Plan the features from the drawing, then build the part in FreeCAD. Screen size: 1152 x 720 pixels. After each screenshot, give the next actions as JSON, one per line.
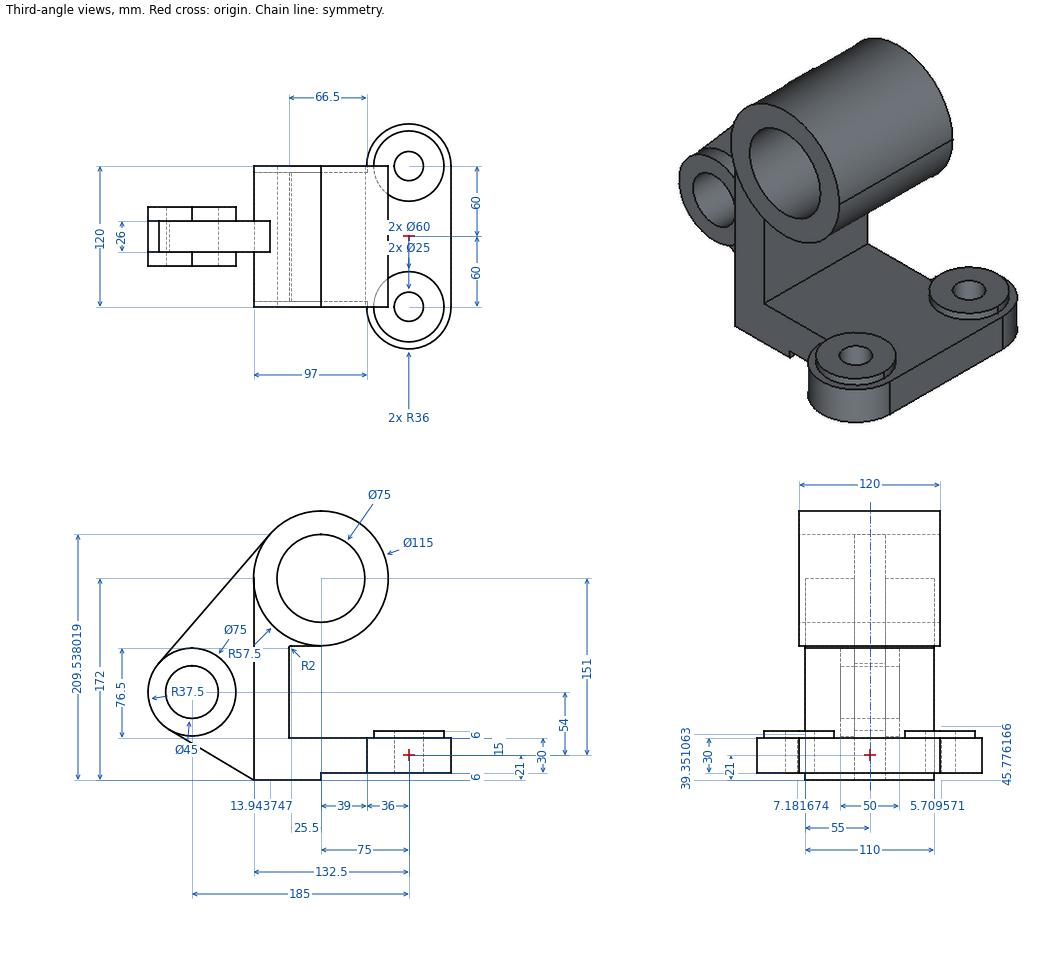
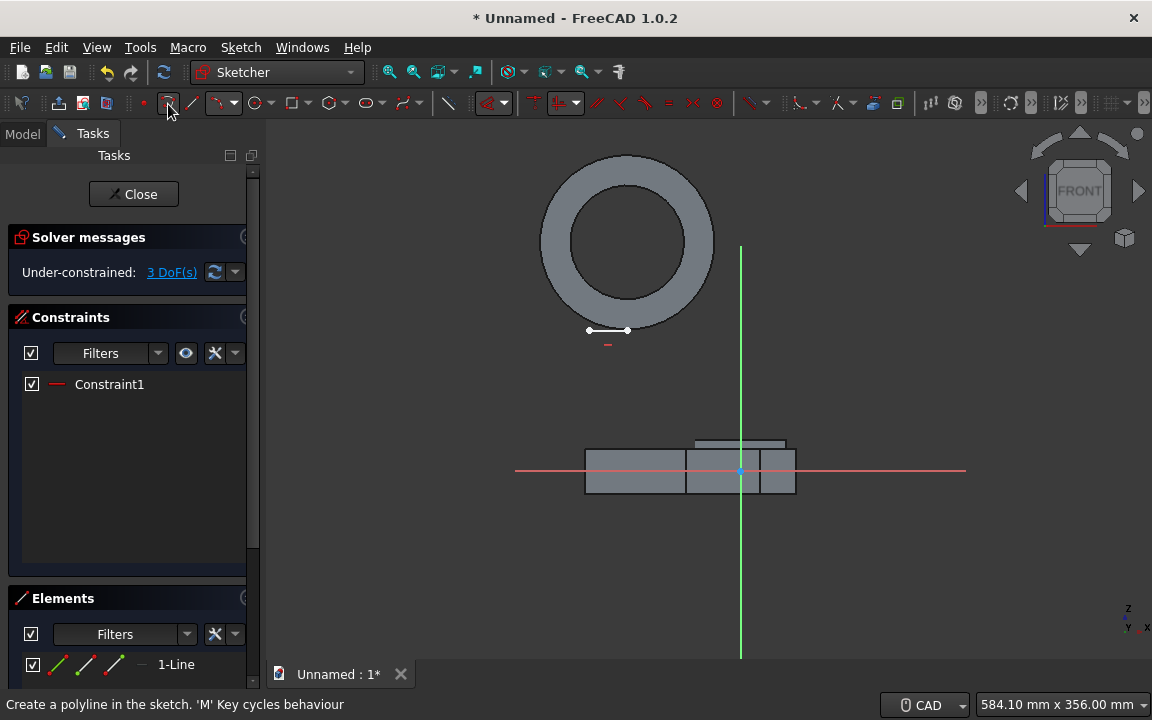
{"action": "scroll", "coordinate": [586, 333], "scroll_direction": "up", "scroll_amount": 7}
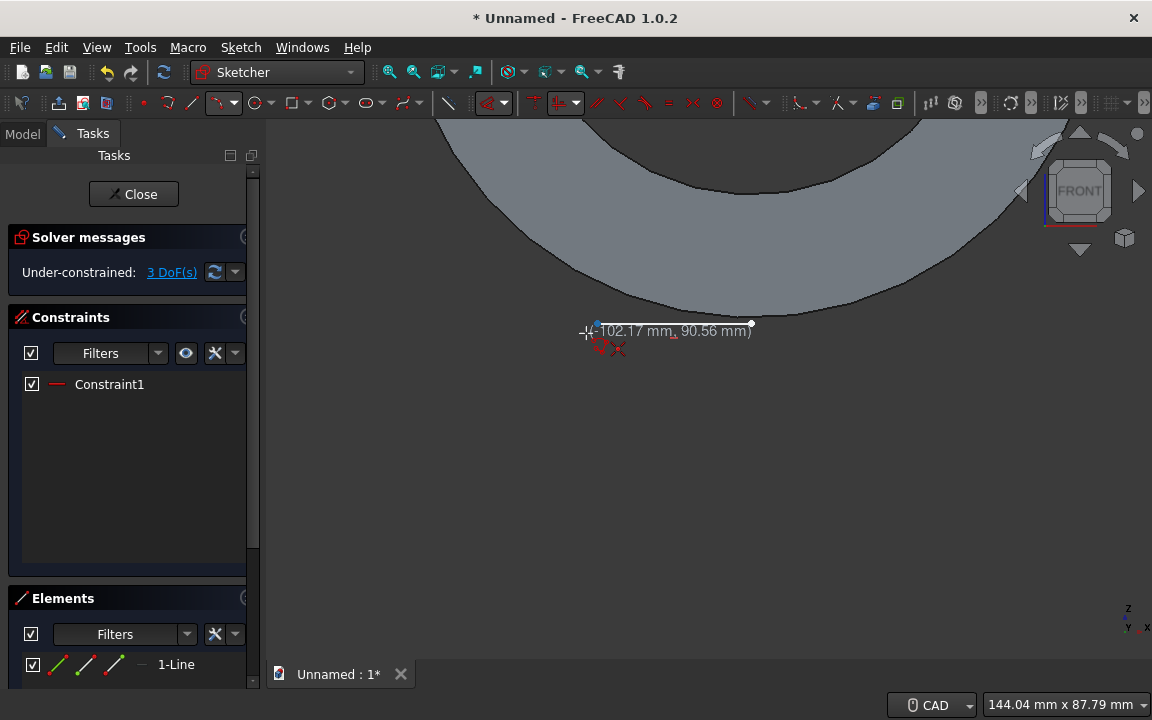
{"action": "left_click", "coordinate": [583, 330]}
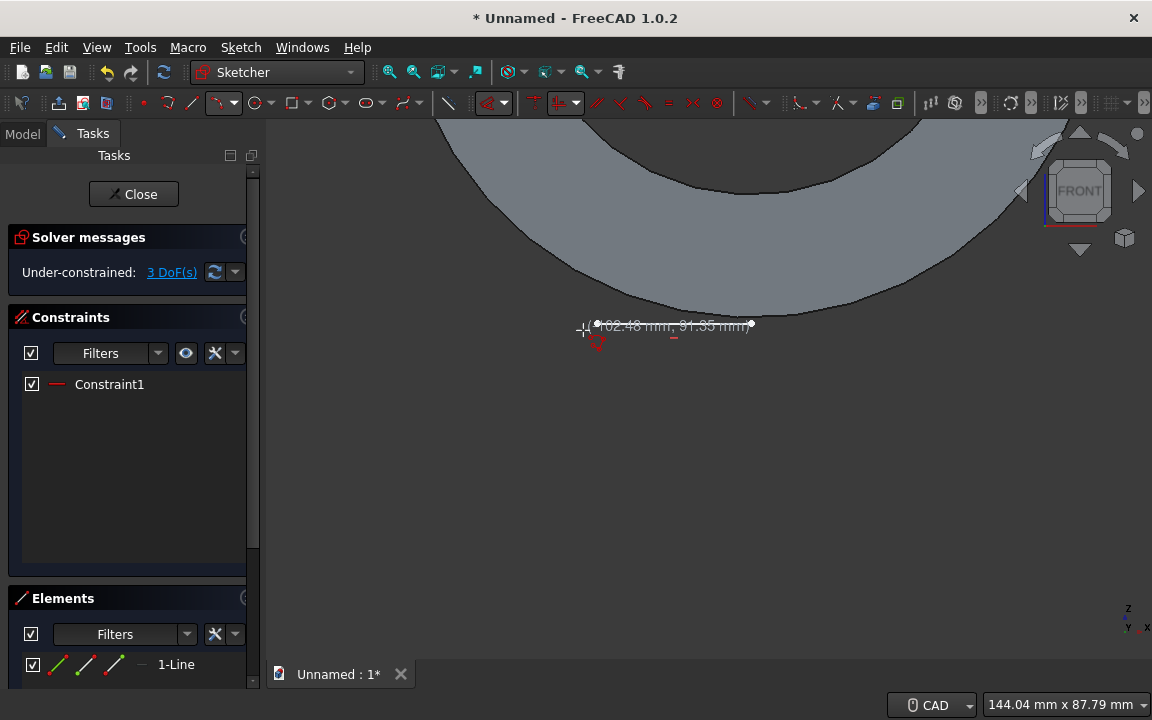
{"action": "scroll", "coordinate": [569, 344], "scroll_direction": "down", "scroll_amount": 6}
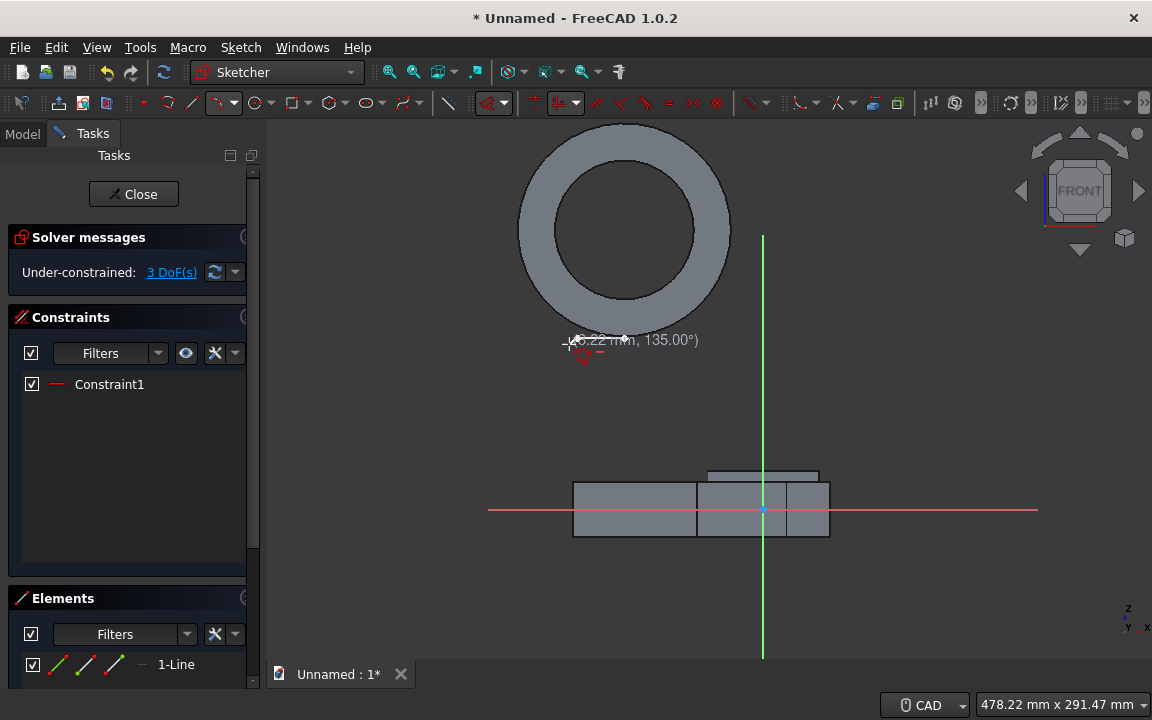
{"action": "left_click", "coordinate": [573, 482]}
{"action": "left_click", "coordinate": [697, 482]}
{"action": "left_click", "coordinate": [697, 537]}
{"action": "left_click", "coordinate": [624, 537]}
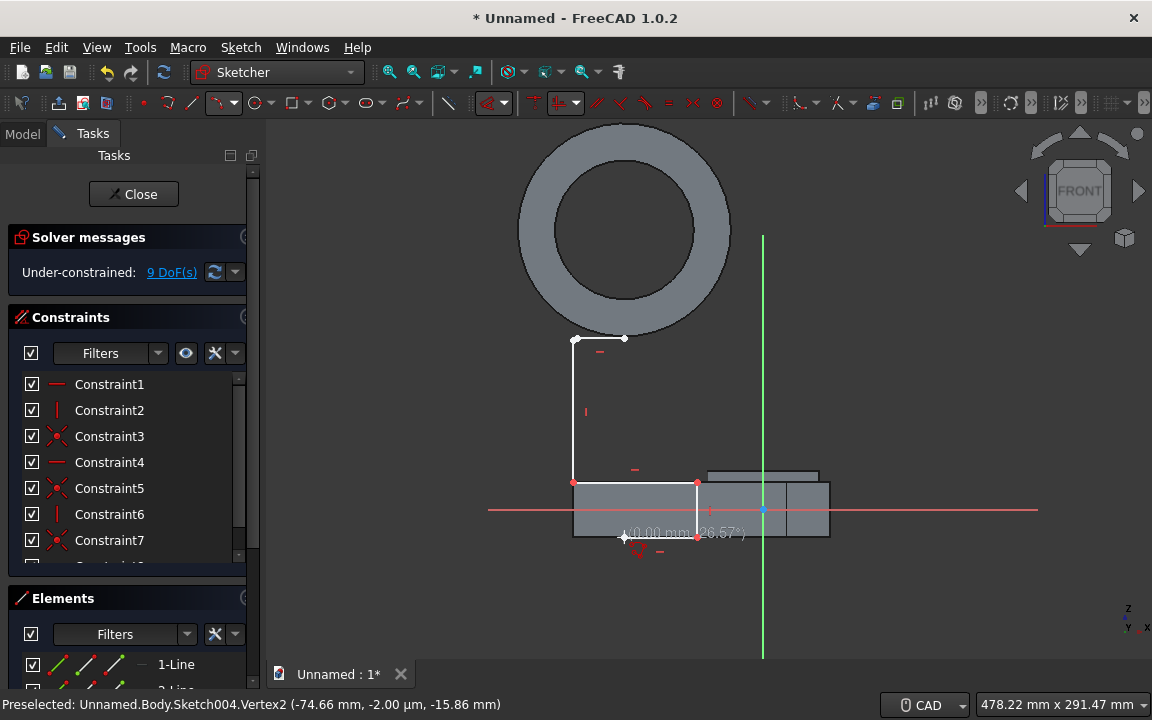
{"action": "scroll", "coordinate": [624, 549], "scroll_direction": "up", "scroll_amount": 2}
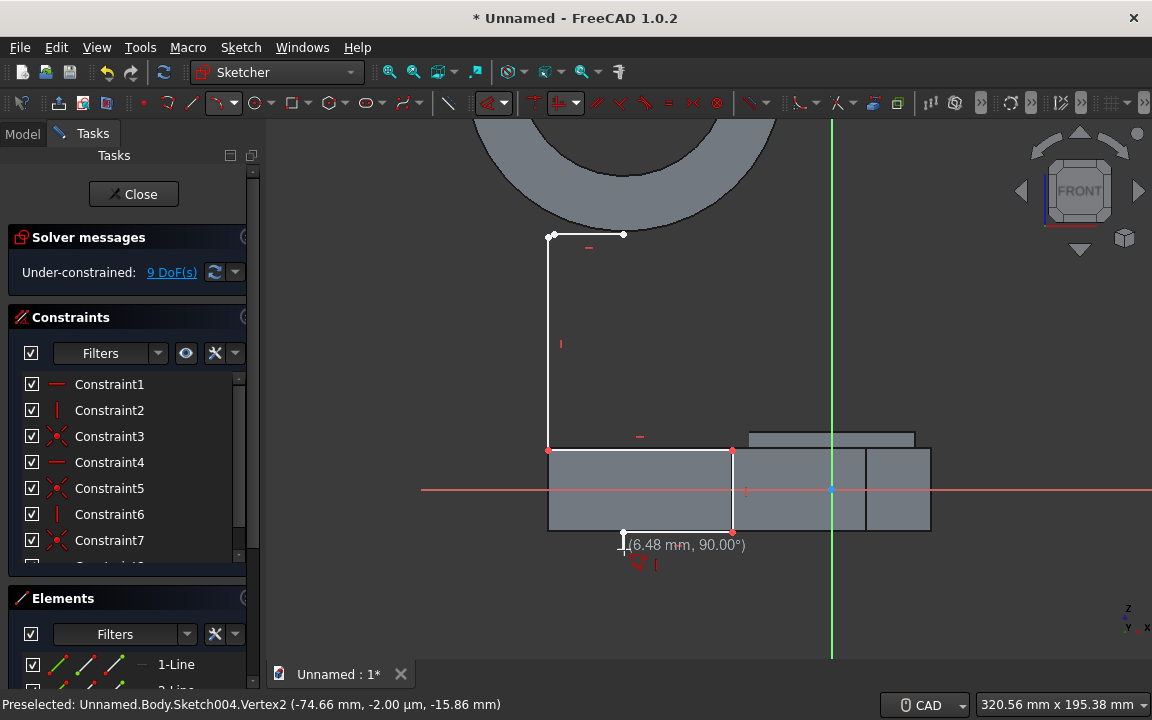
{"action": "left_click", "coordinate": [624, 548]}
{"action": "left_click", "coordinate": [465, 548]}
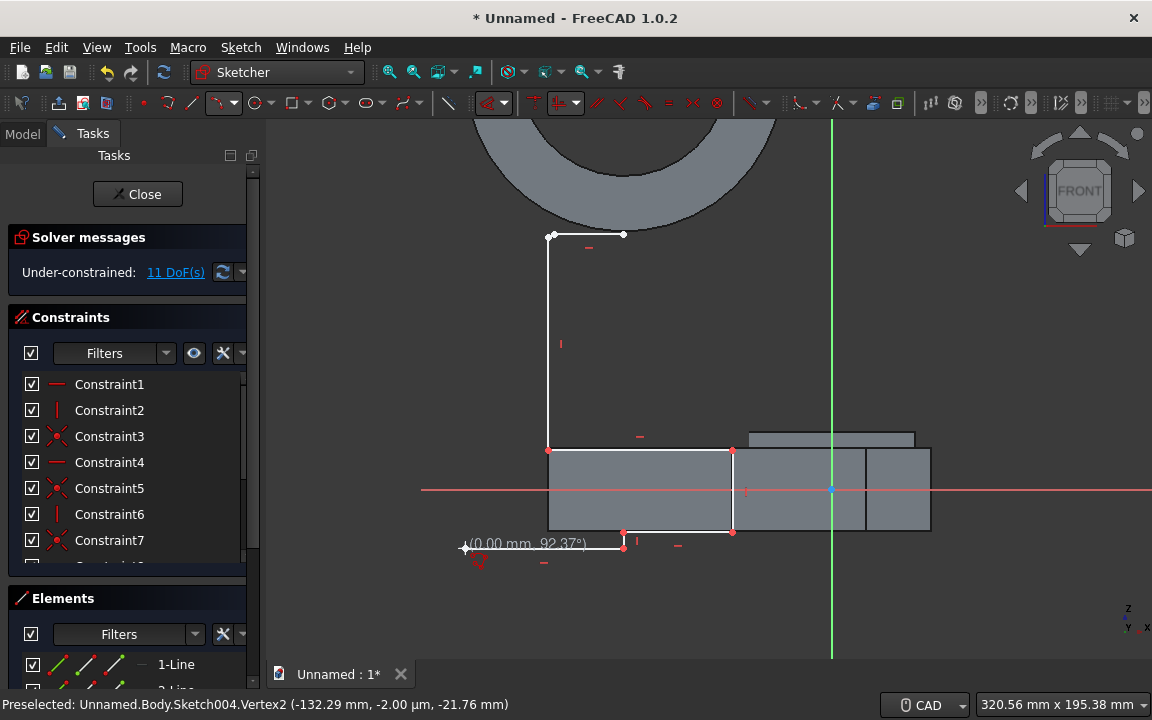
{"action": "scroll", "coordinate": [624, 549], "scroll_direction": "down", "scroll_amount": 2}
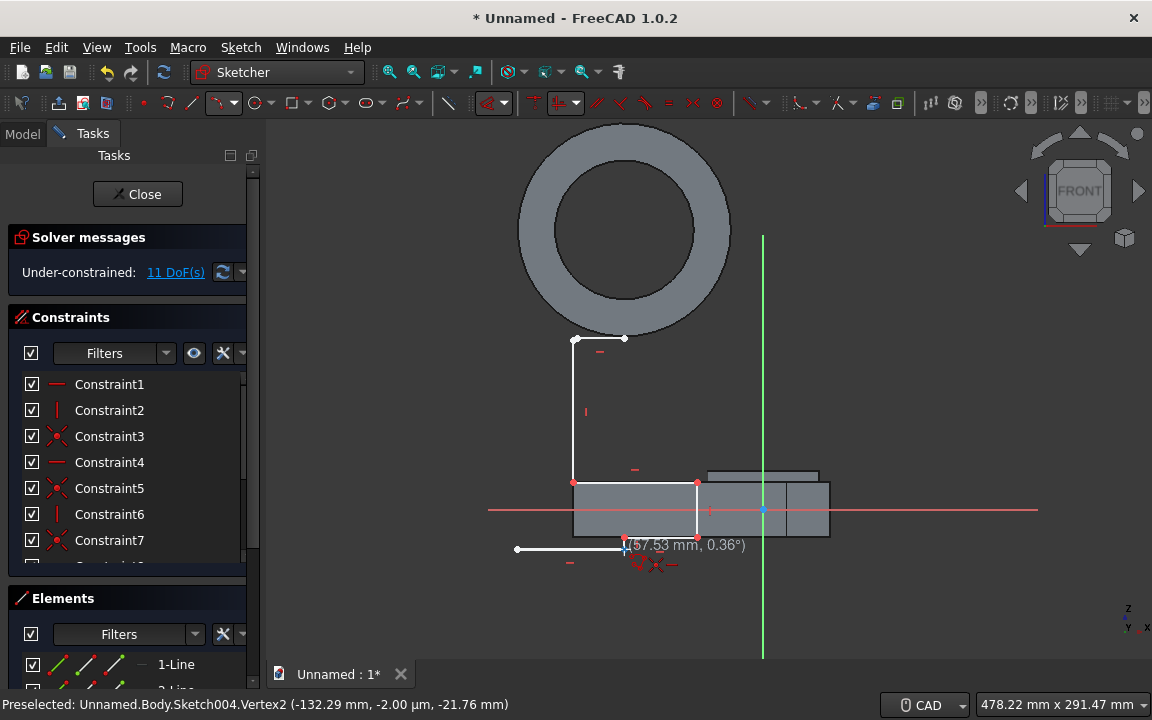
{"action": "left_click", "coordinate": [518, 230]}
{"action": "right_click", "coordinate": [518, 230]}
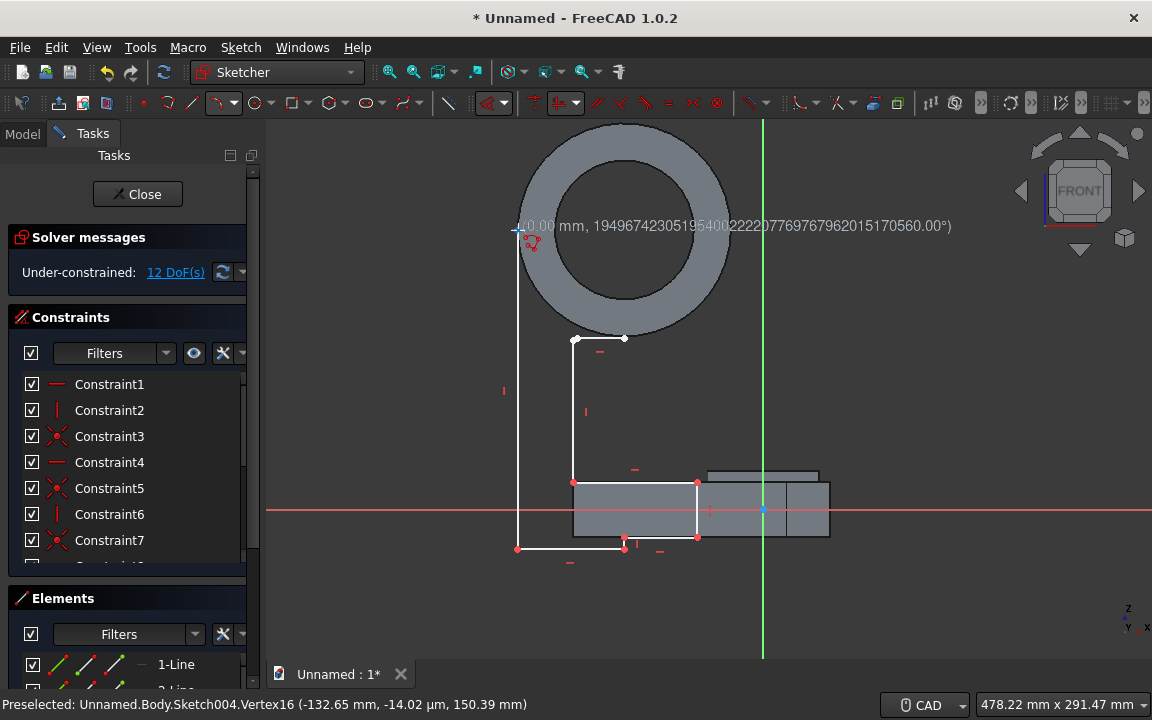
{"action": "key", "text": "g 3 a"}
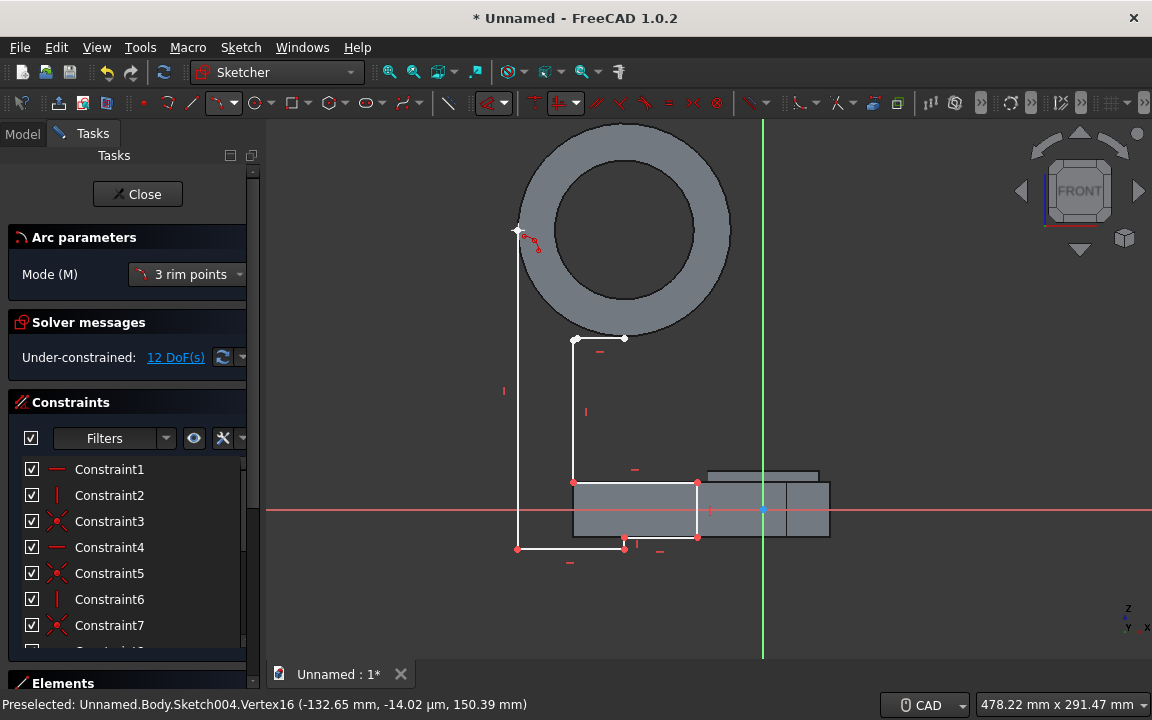
{"action": "scroll", "coordinate": [577, 336], "scroll_direction": "up", "scroll_amount": 6}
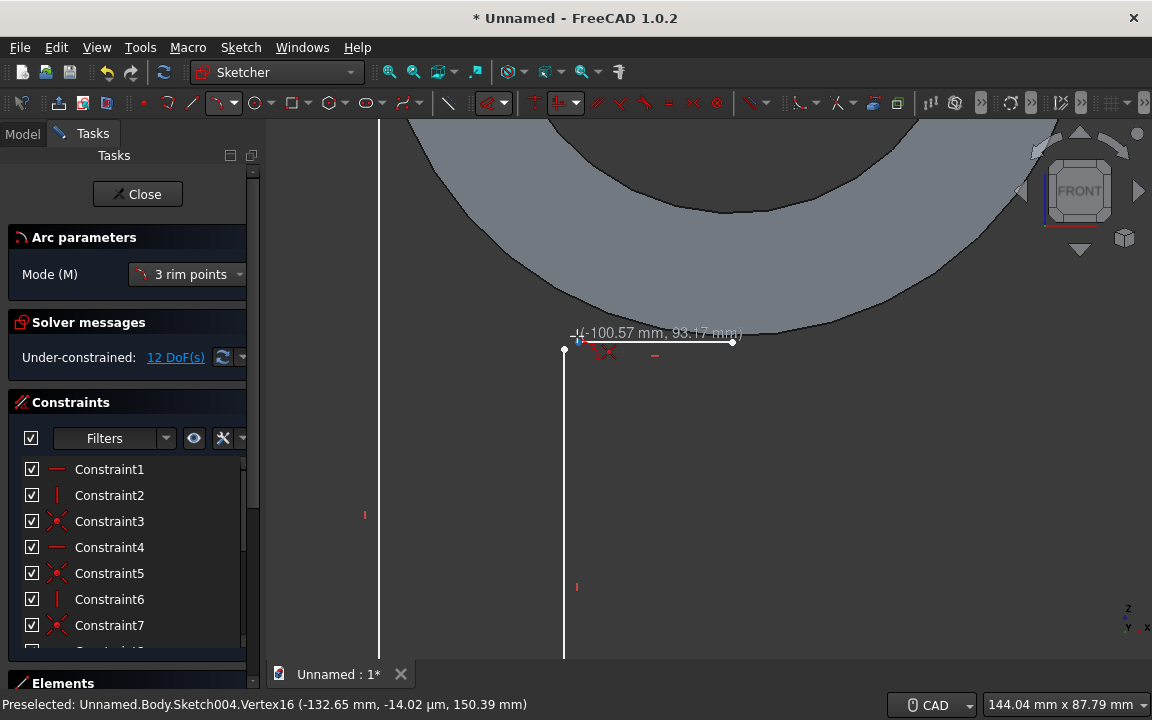
{"action": "left_click", "coordinate": [578, 342]}
{"action": "left_click", "coordinate": [564, 350]}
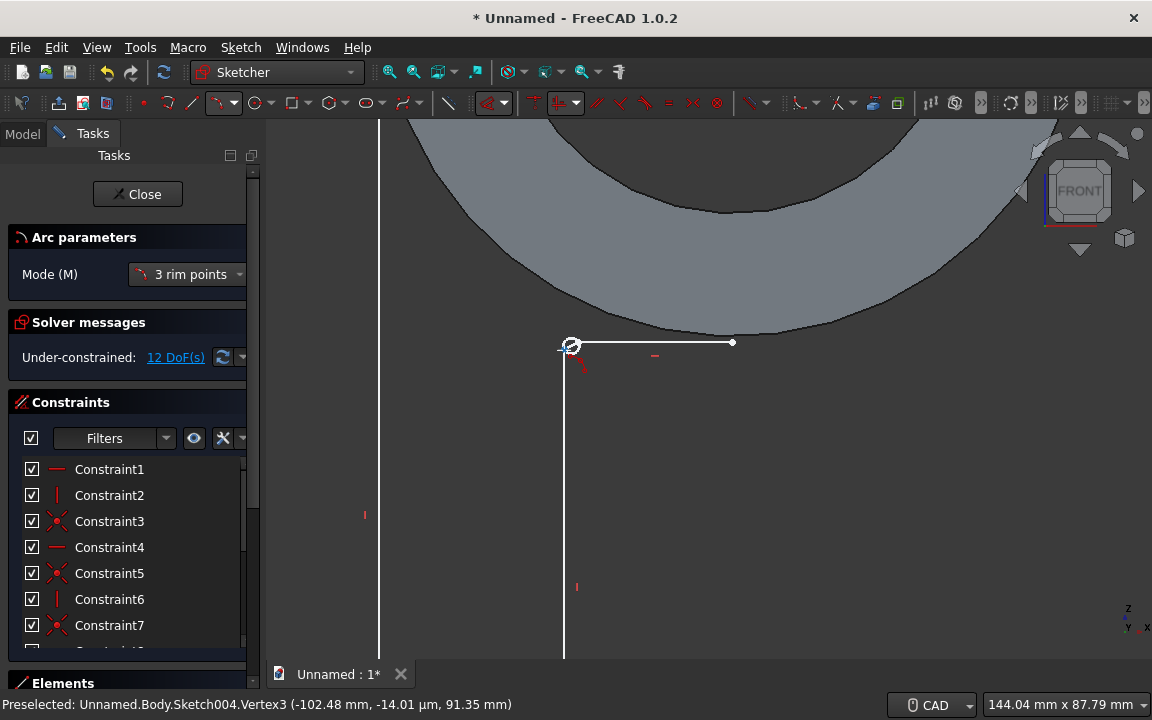
{"action": "scroll", "coordinate": [568, 340], "scroll_direction": "up", "scroll_amount": 8}